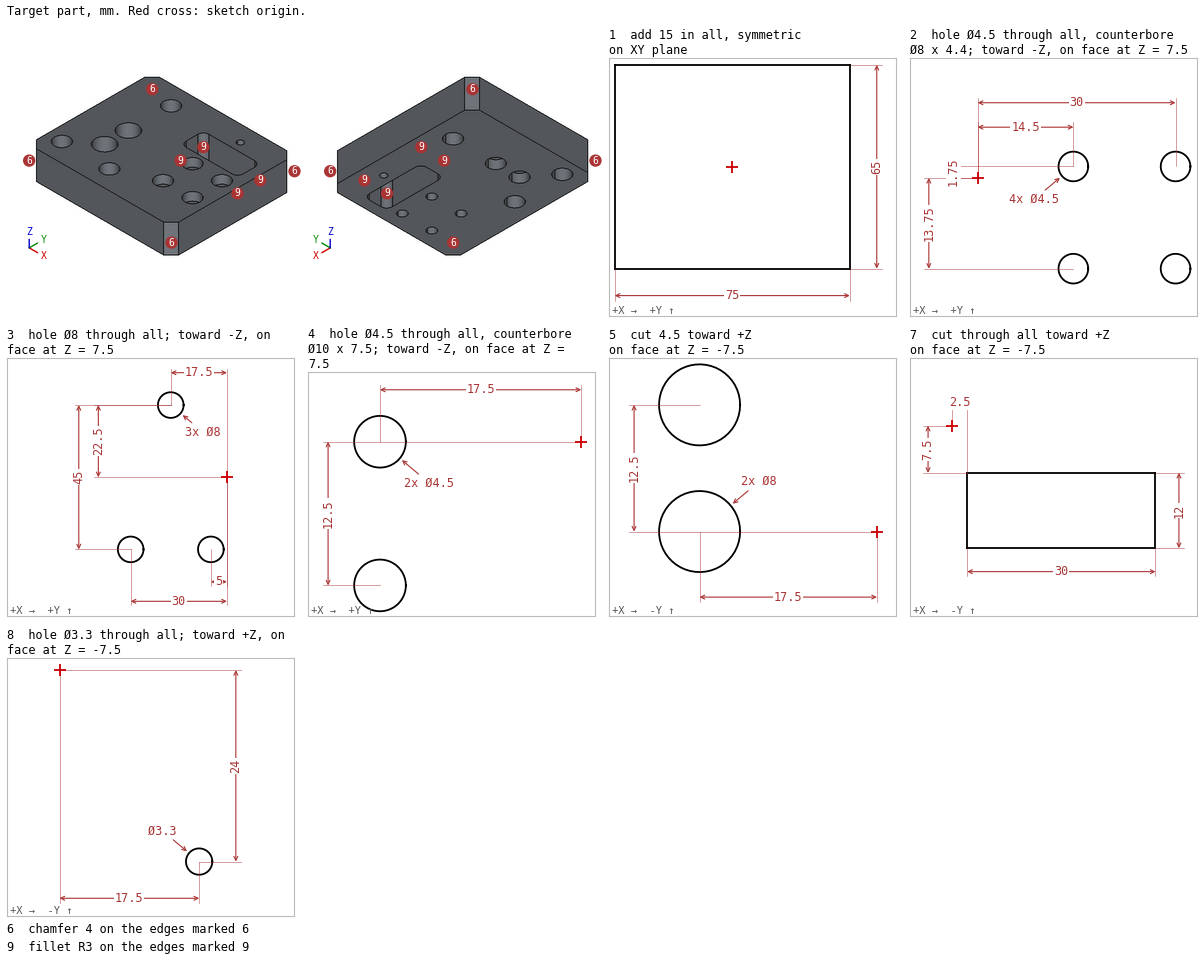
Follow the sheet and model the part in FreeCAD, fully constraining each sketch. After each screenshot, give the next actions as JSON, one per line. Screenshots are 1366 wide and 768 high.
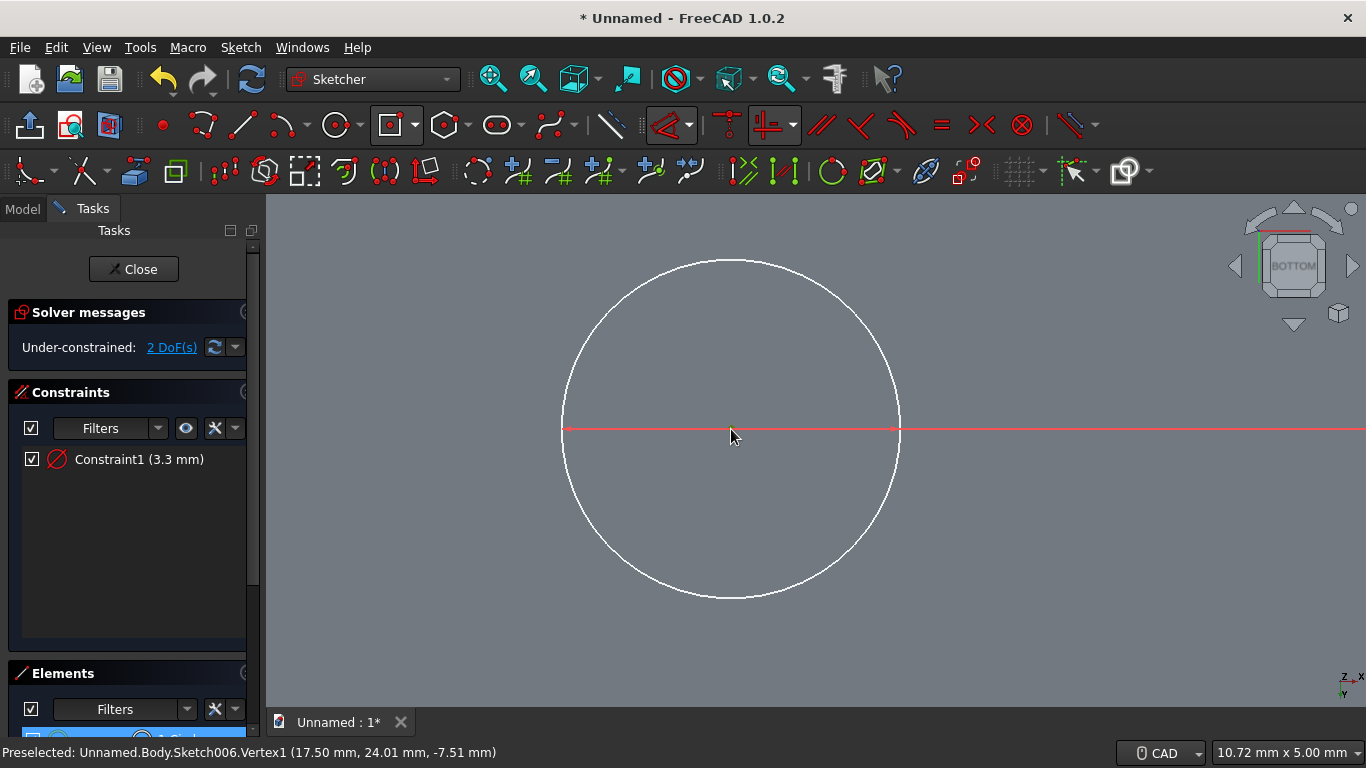
{"action": "left_click", "coordinate": [692, 126]}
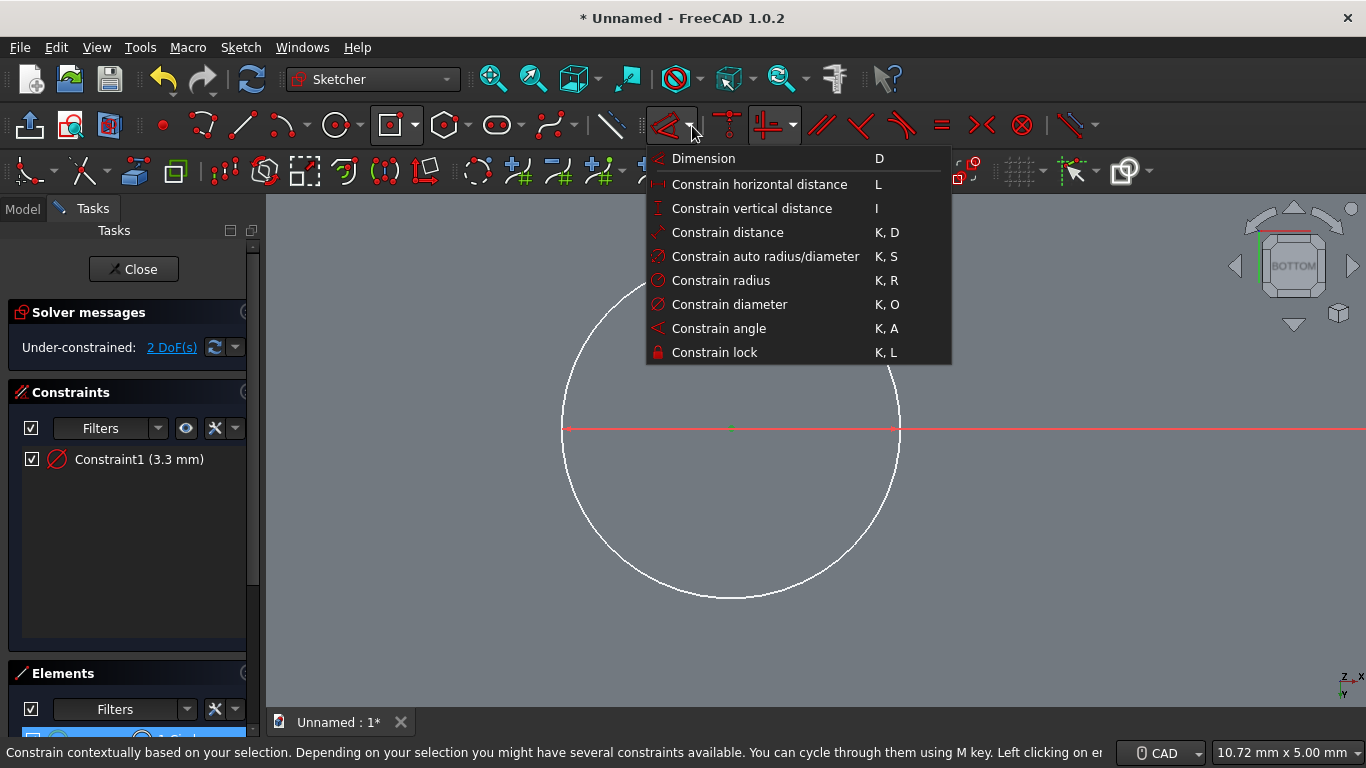
{"action": "left_click", "coordinate": [799, 208]}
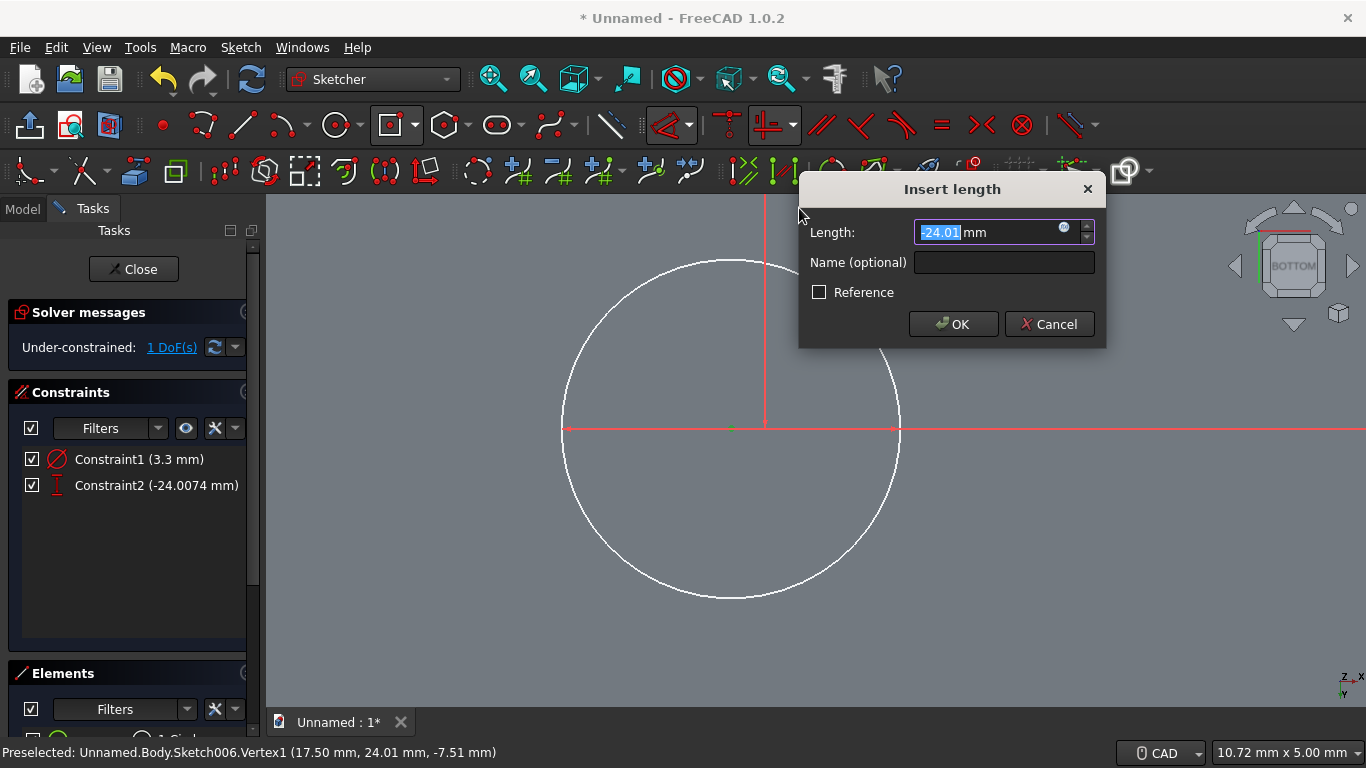
{"action": "type", "text": "-24"}
{"action": "key", "text": "Return"}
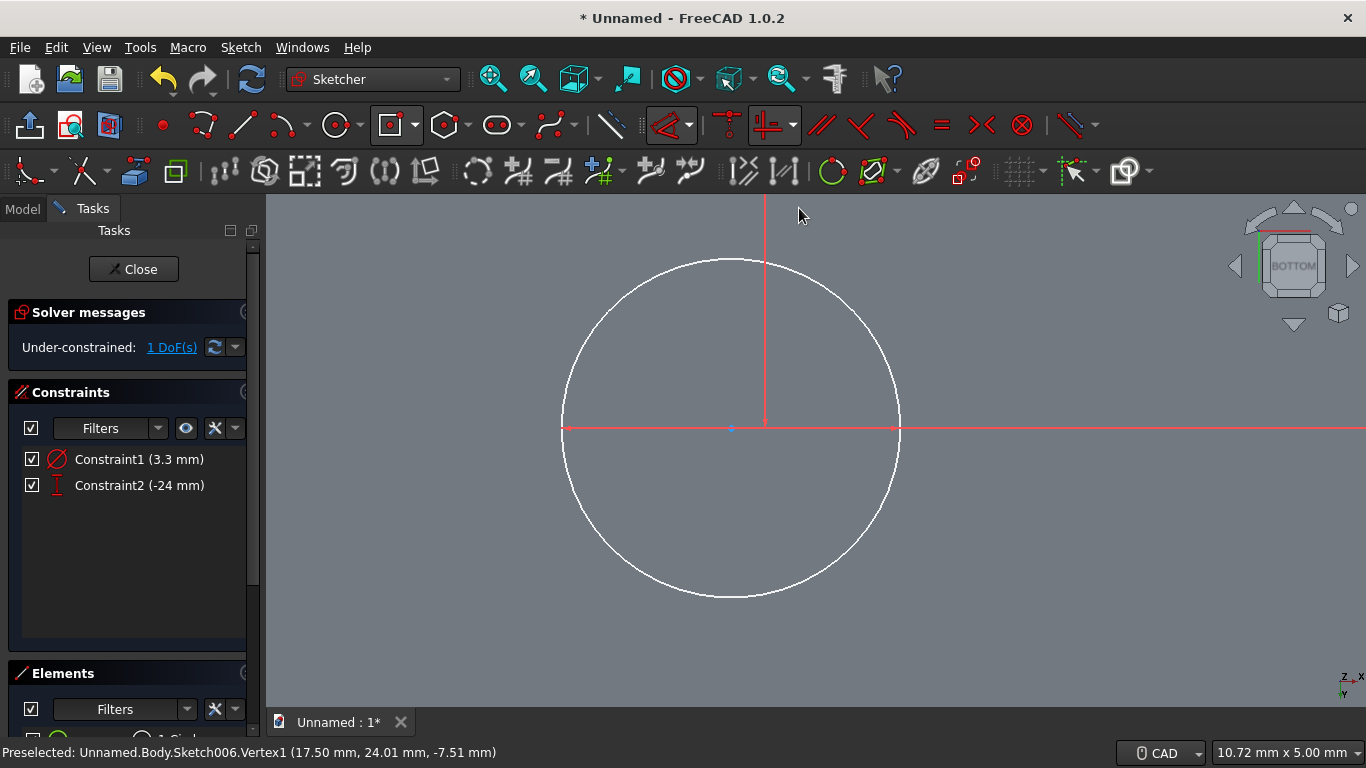
{"action": "left_click", "coordinate": [731, 428]}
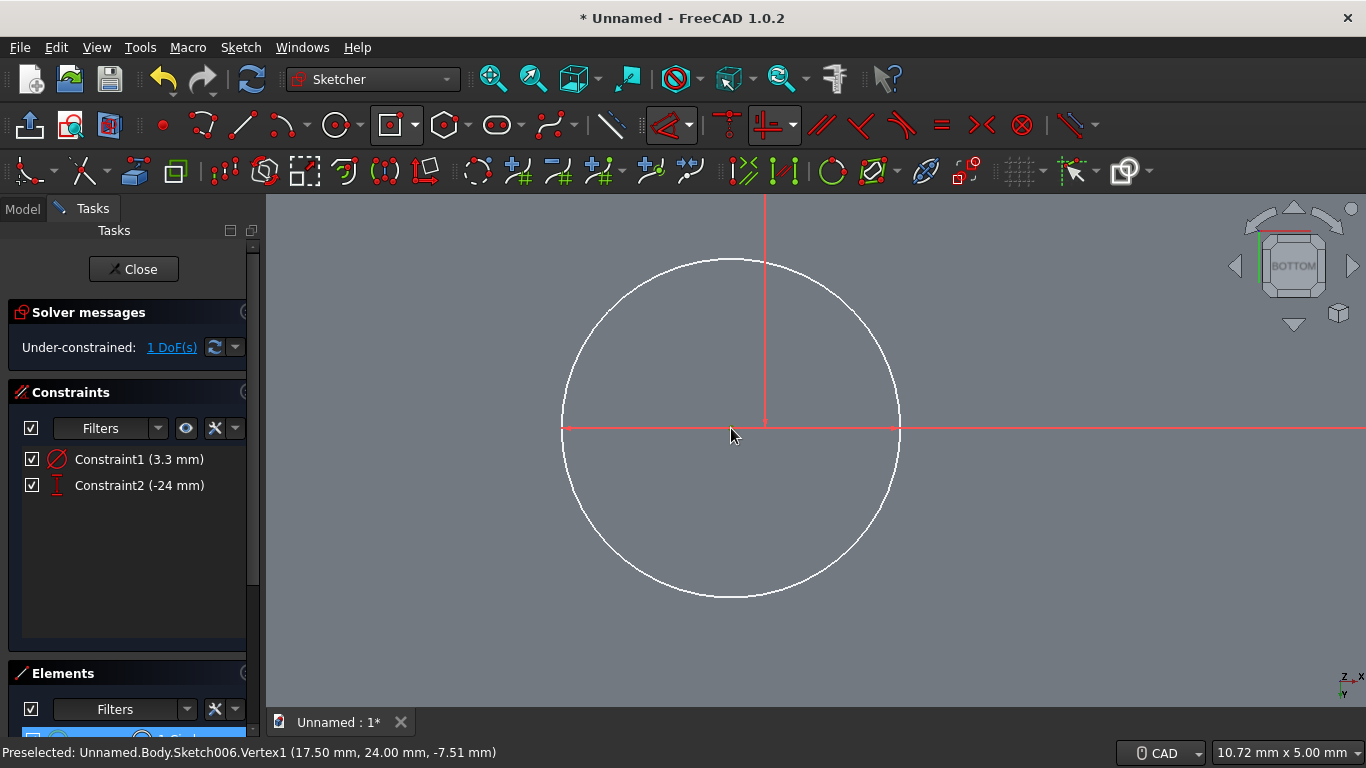
{"action": "key", "text": "l"}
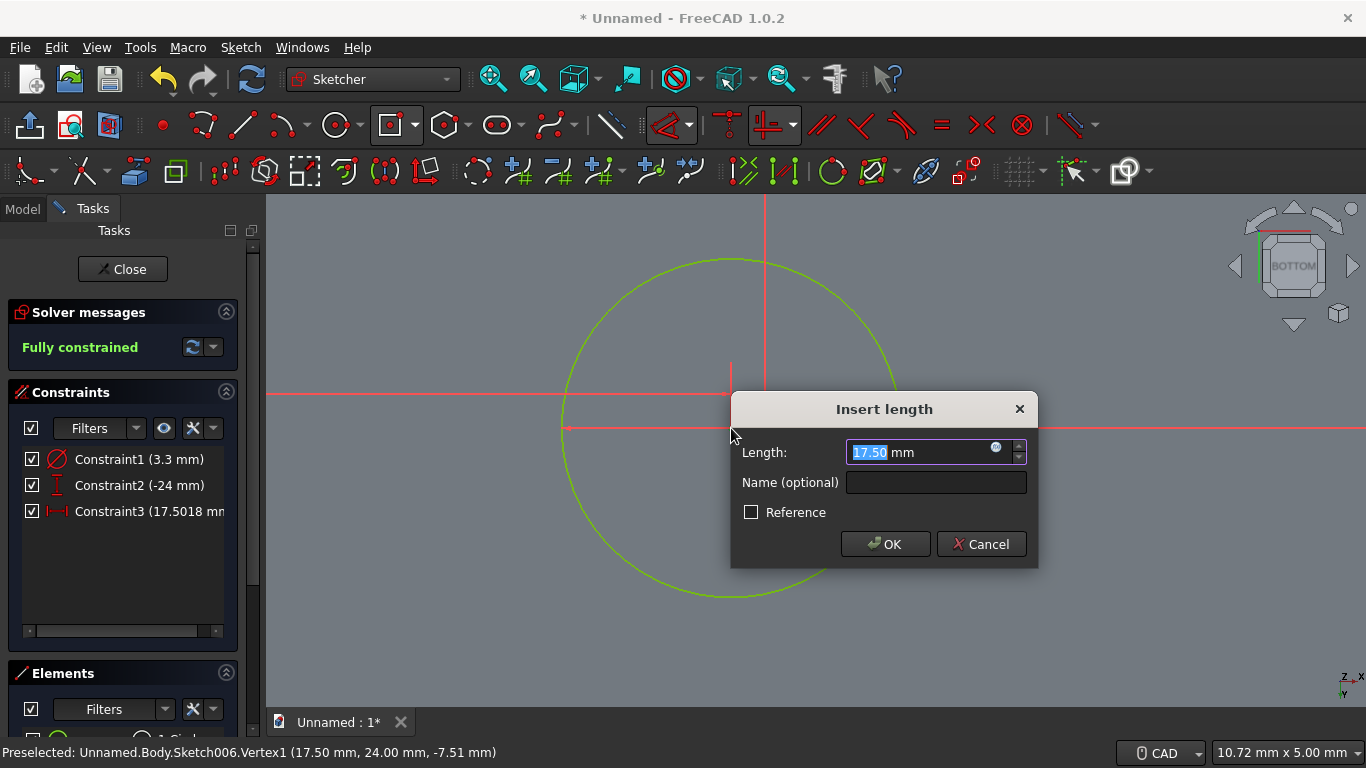
{"action": "type", "text": "17.5"}
{"action": "key", "text": "Return"}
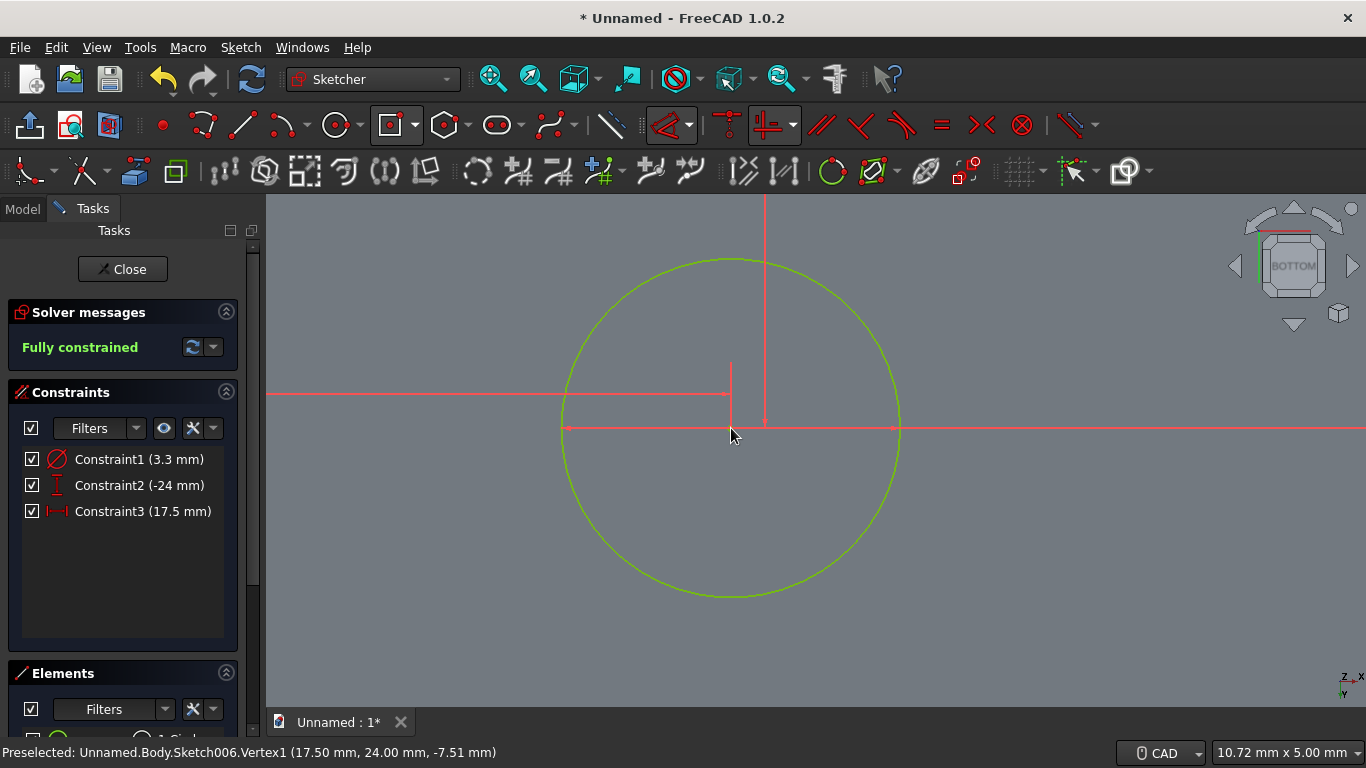
{"action": "left_click", "coordinate": [123, 269]}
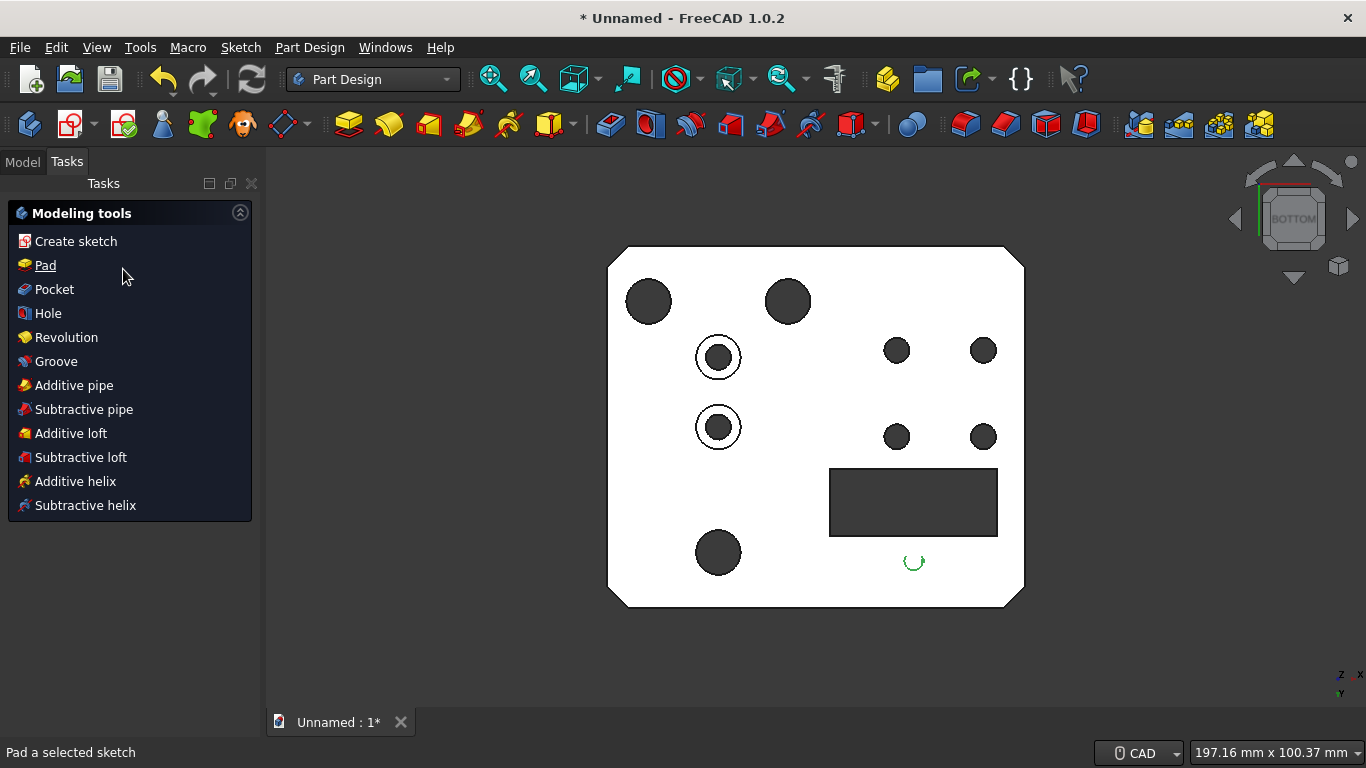
{"action": "left_click", "coordinate": [652, 124]}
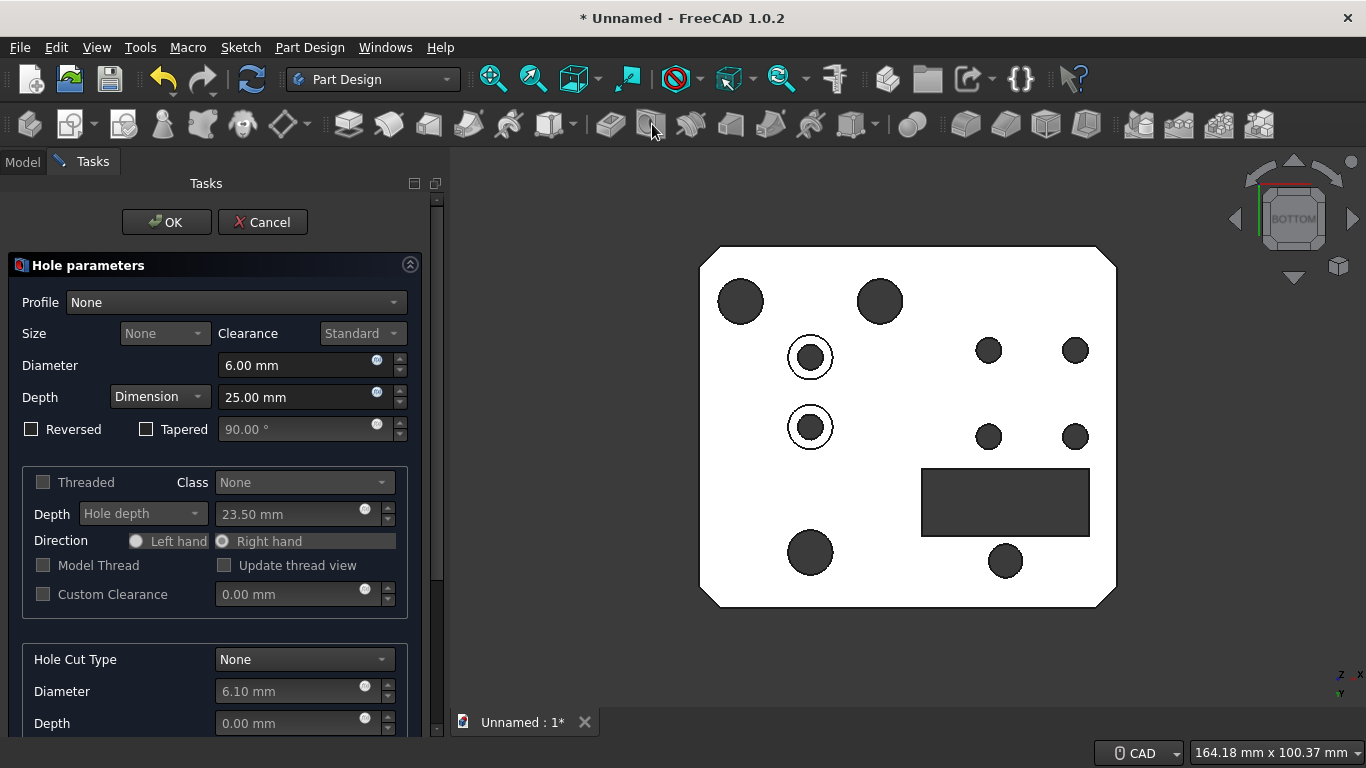
{"action": "triple_click", "coordinate": [305, 365]}